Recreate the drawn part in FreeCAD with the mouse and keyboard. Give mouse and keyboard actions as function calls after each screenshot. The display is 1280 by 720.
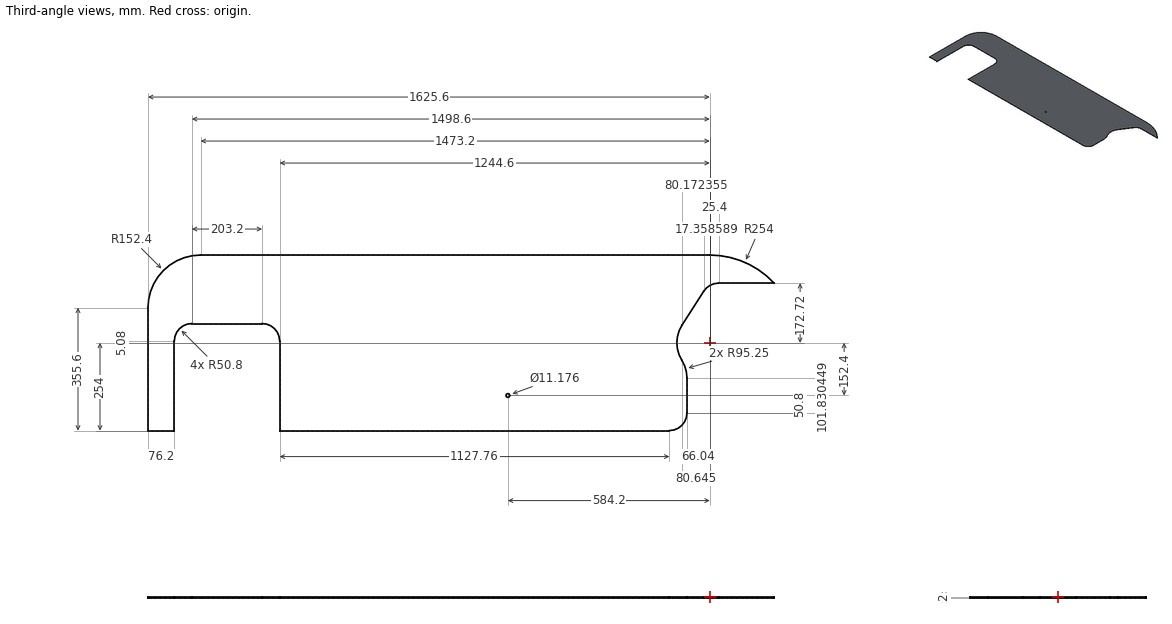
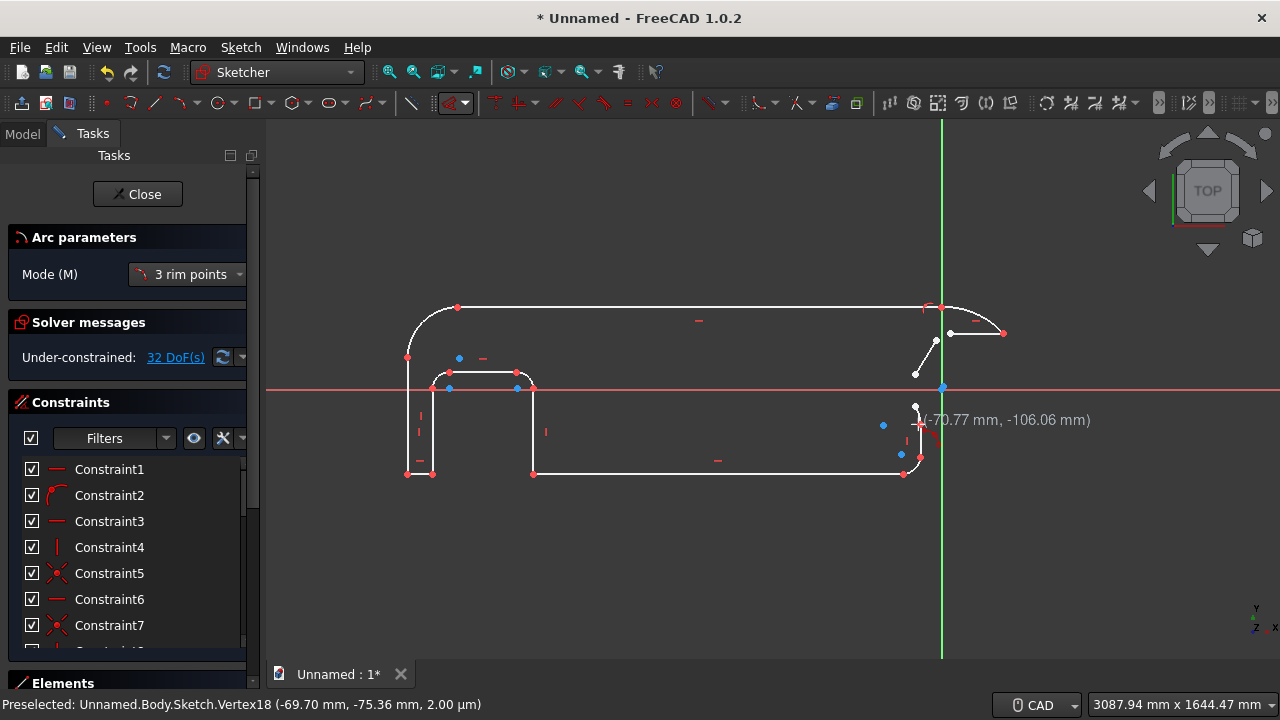
click(915, 407)
click(916, 374)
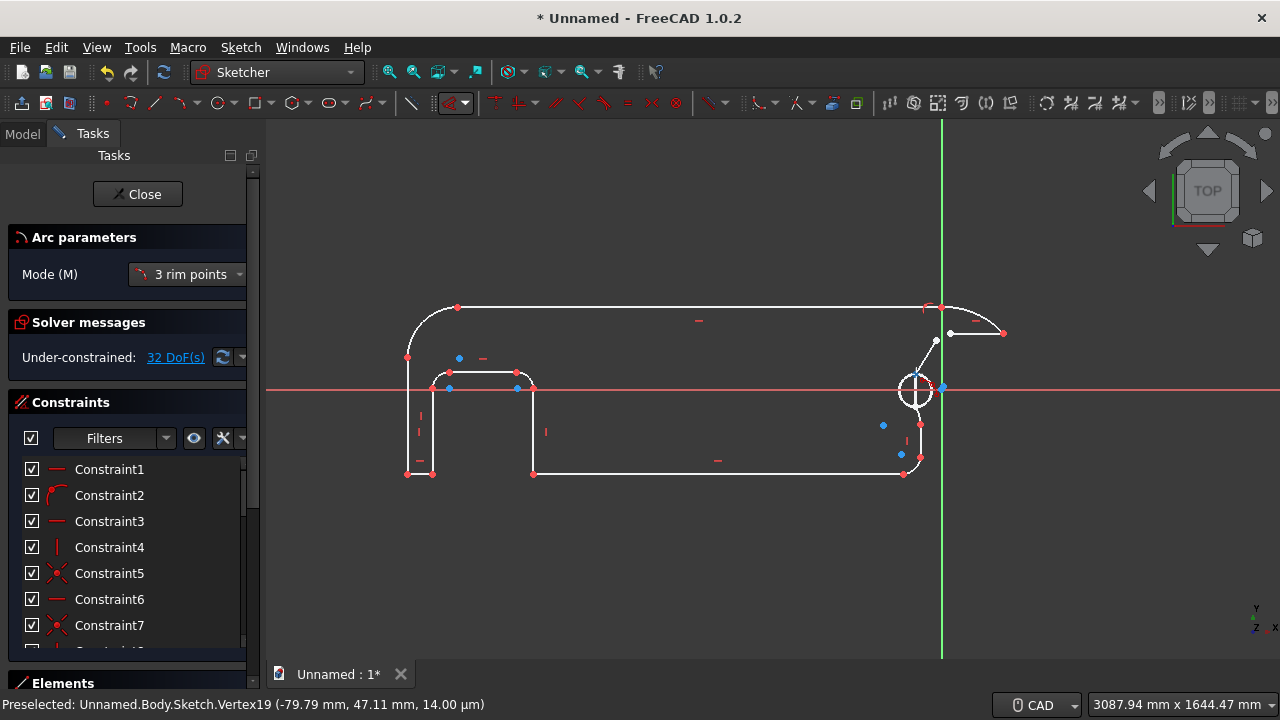
scroll(911, 397, up, 7)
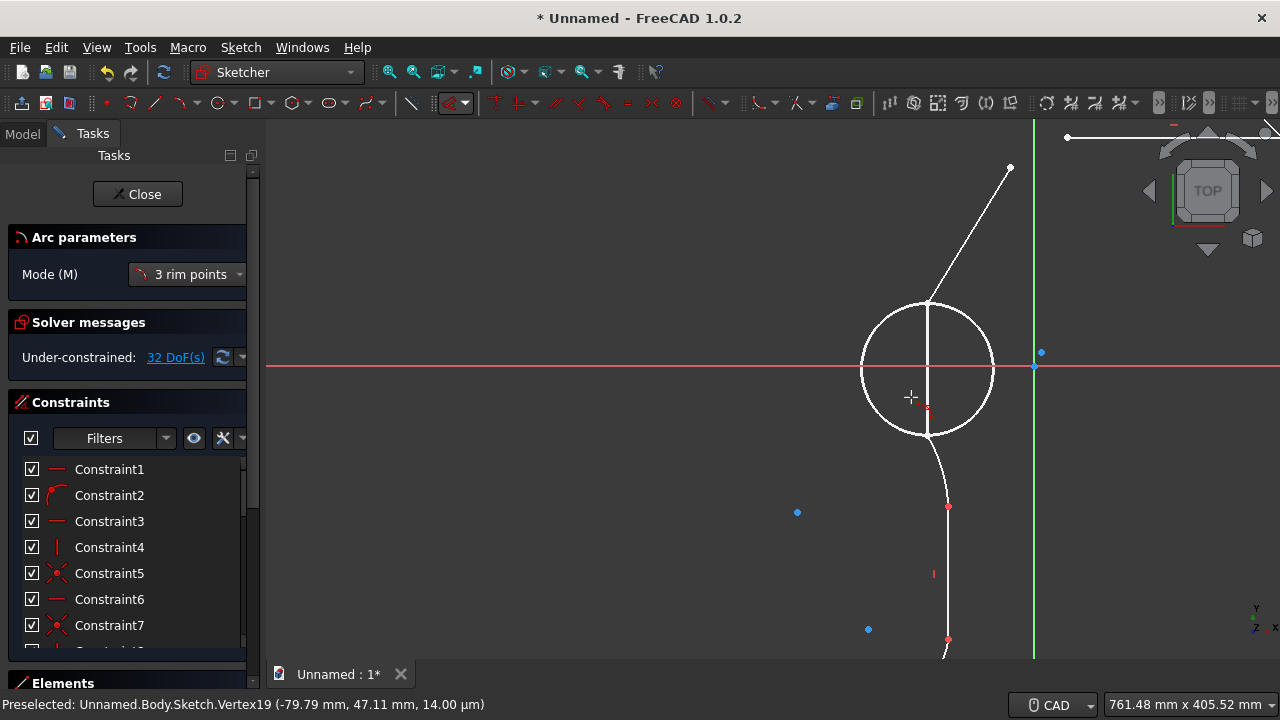
click(910, 394)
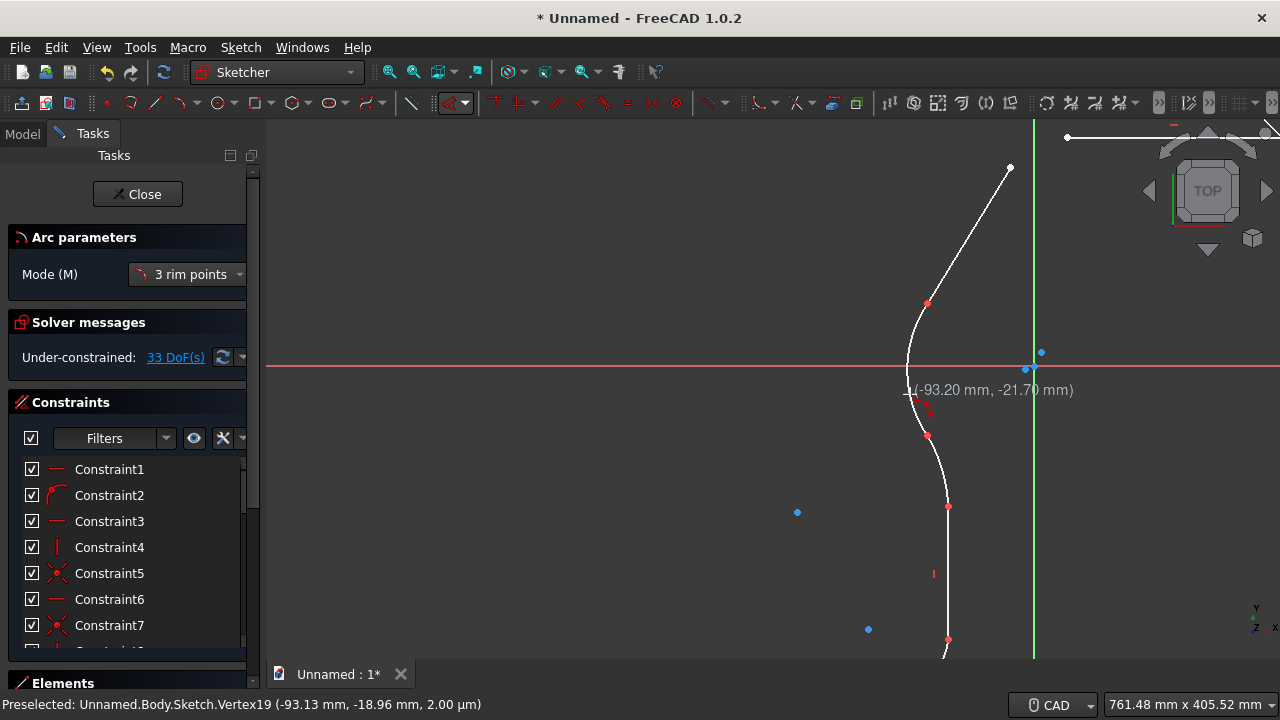
click(1011, 168)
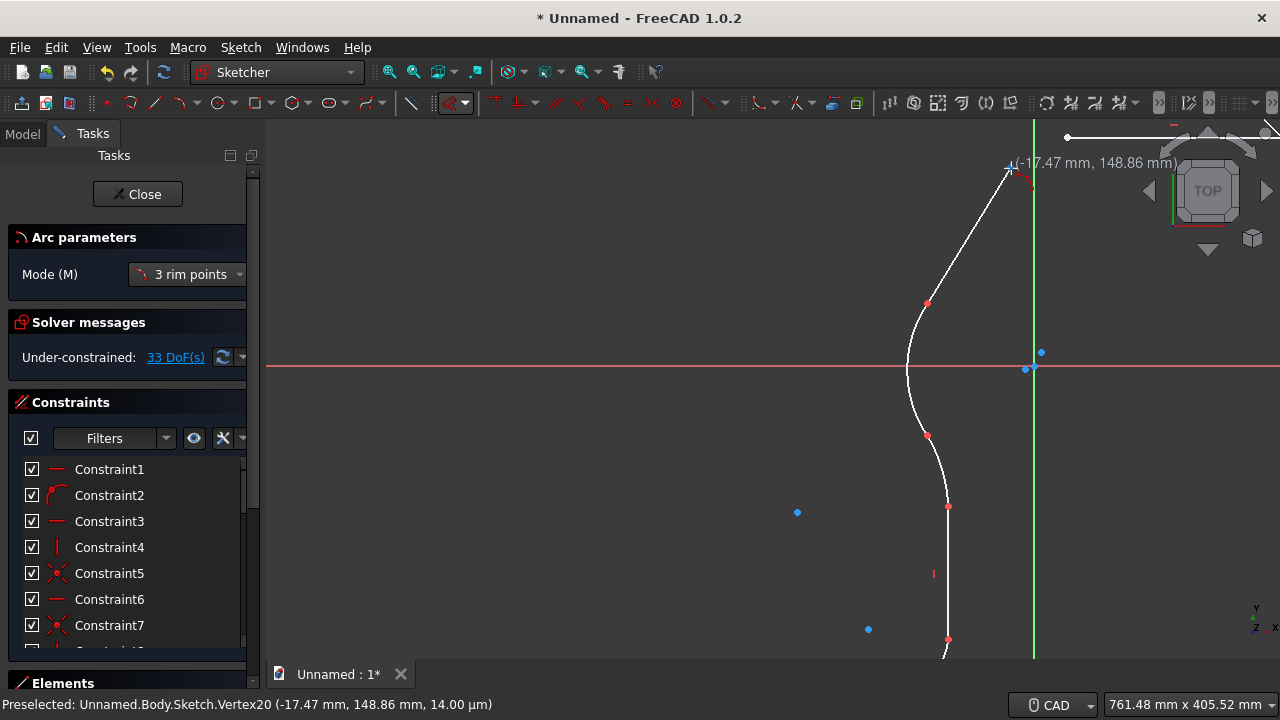
scroll(910, 396, down, 7)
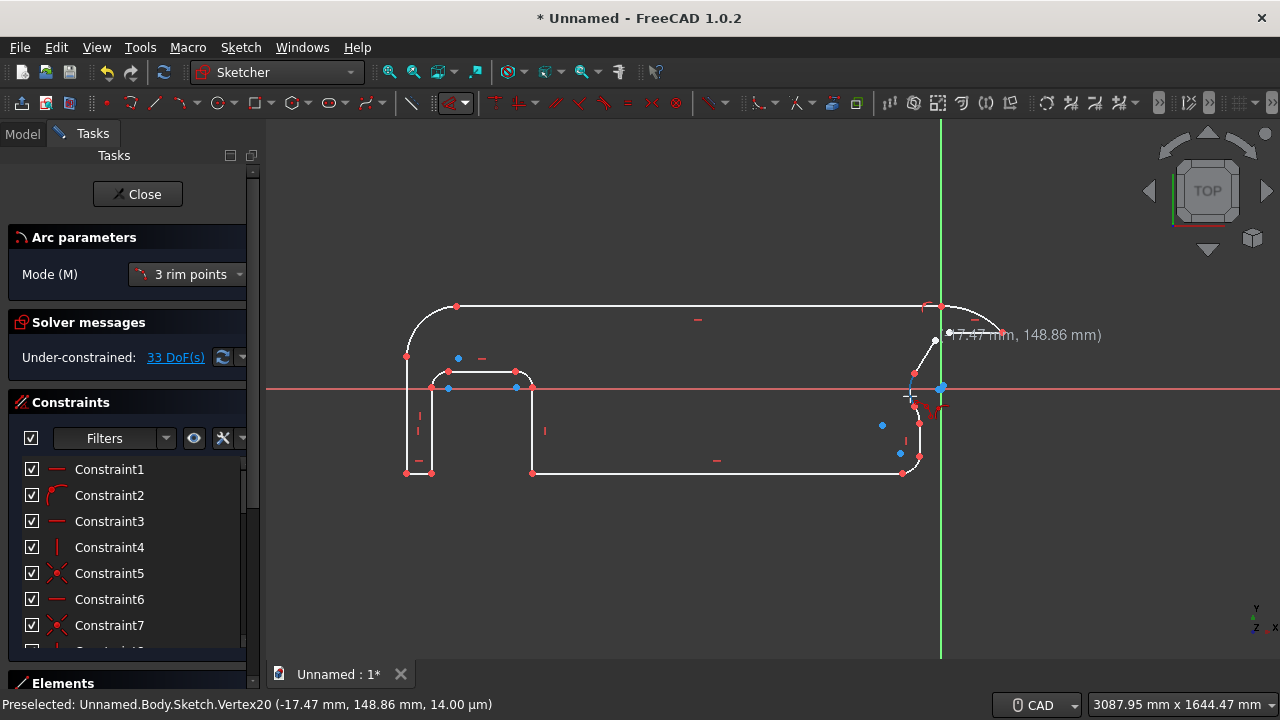
scroll(949, 332, up, 4)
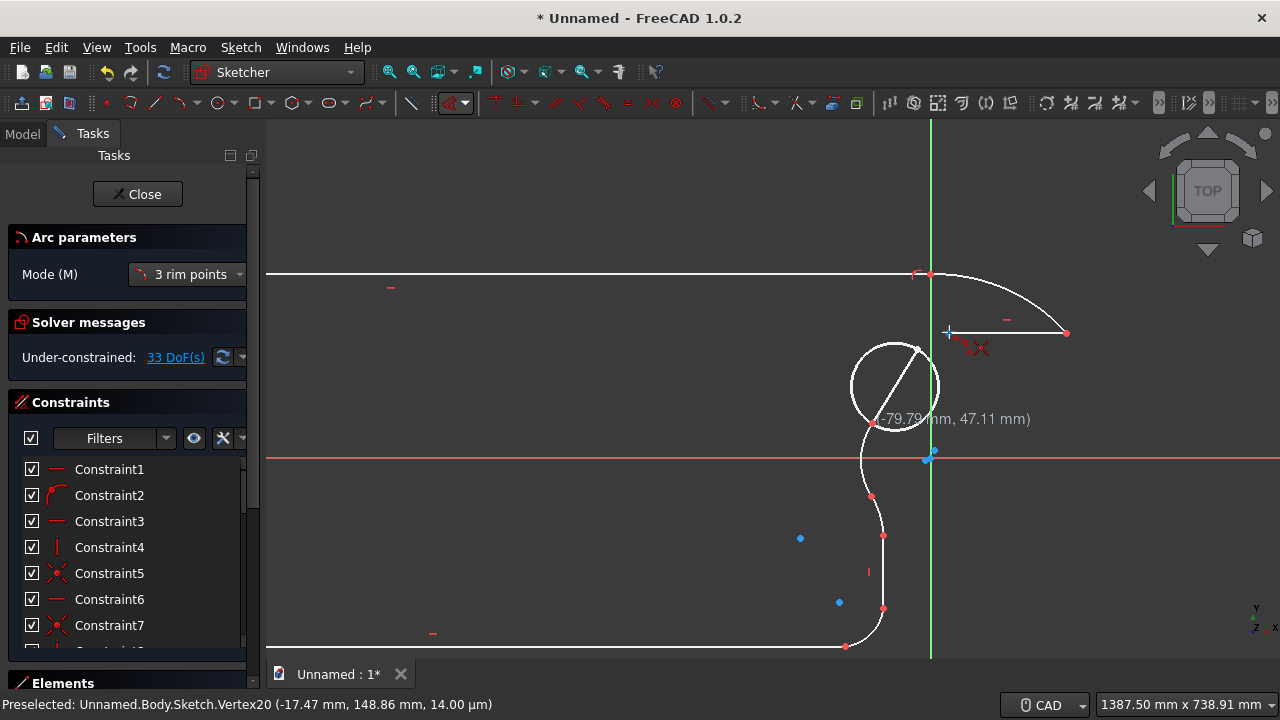
click(949, 333)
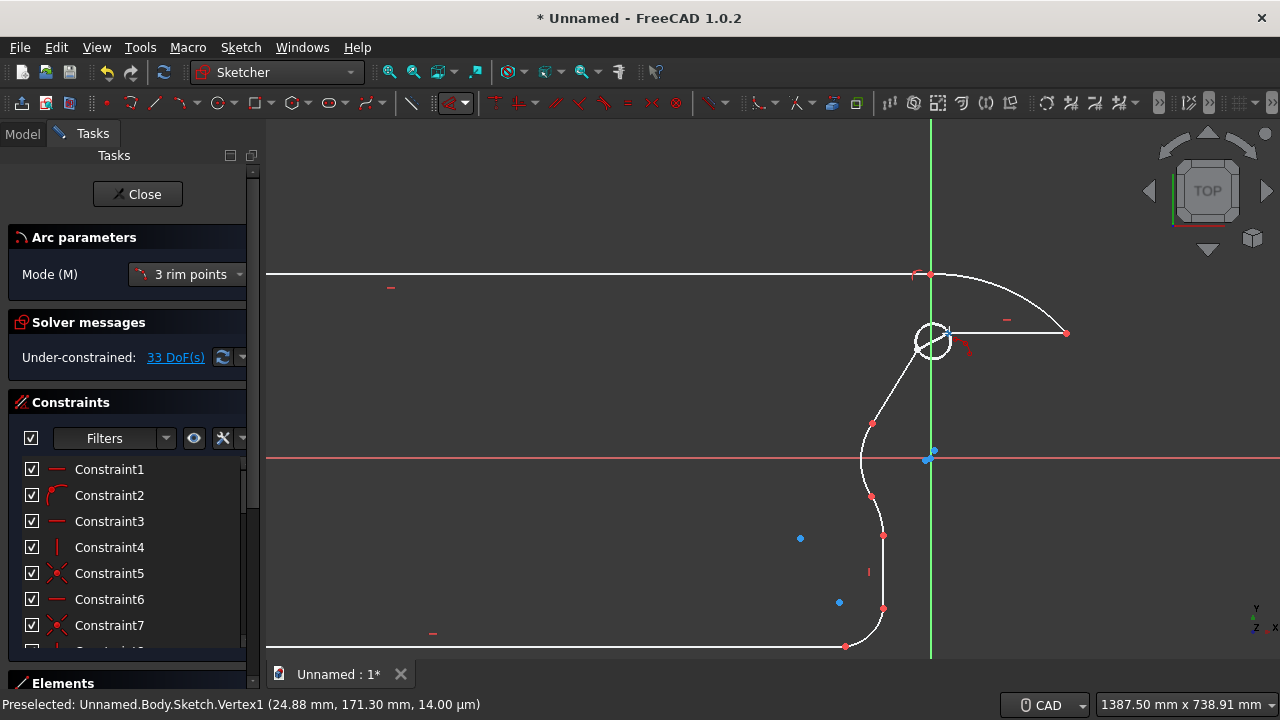
scroll(935, 335, up, 7)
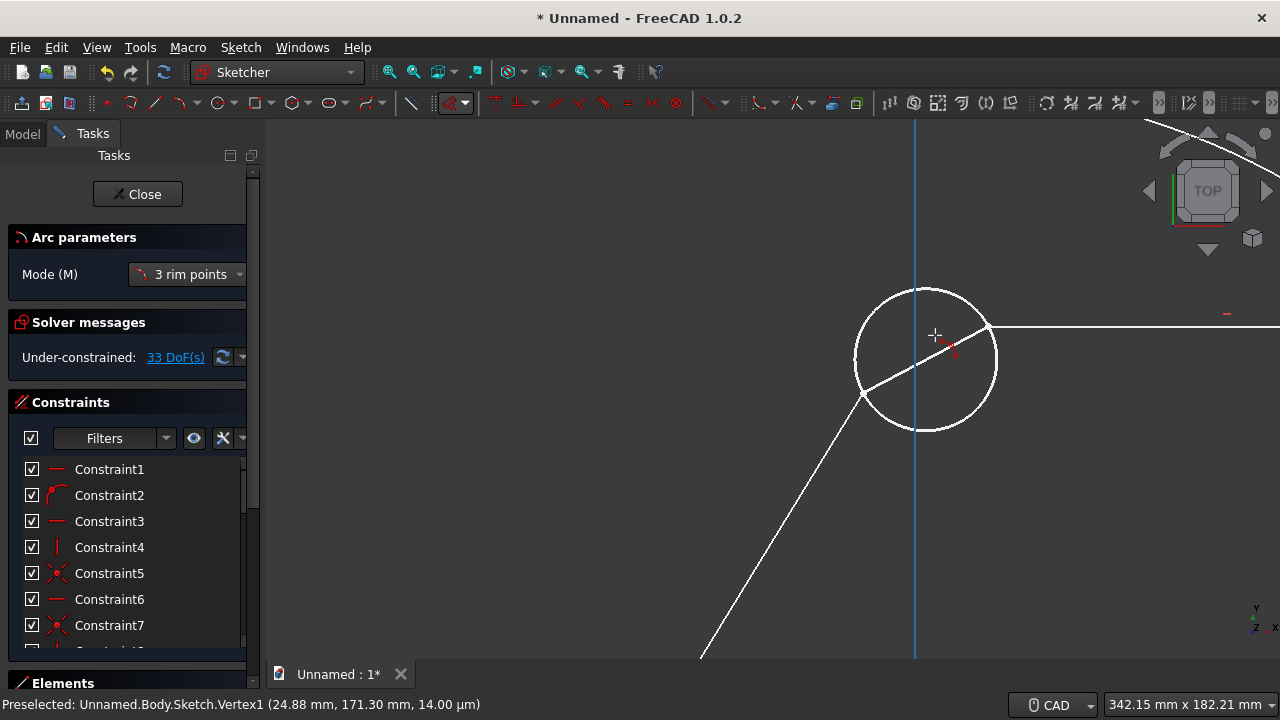
click(932, 334)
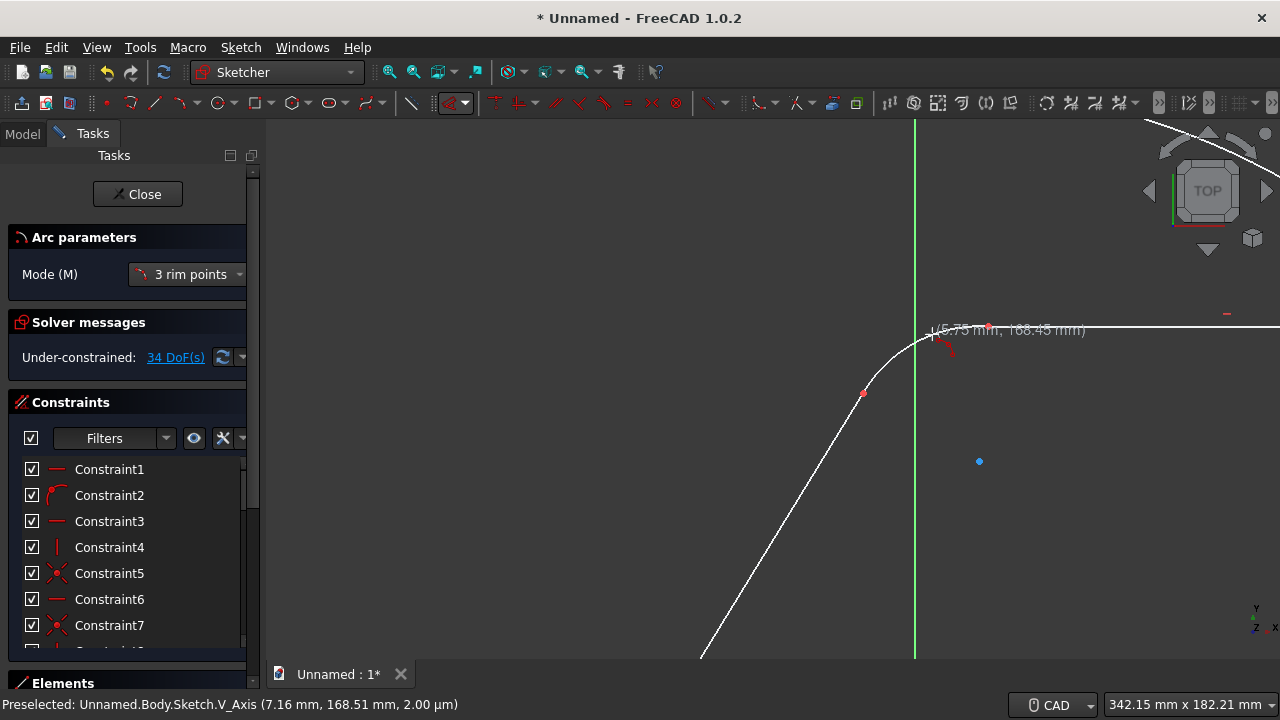
click(218, 104)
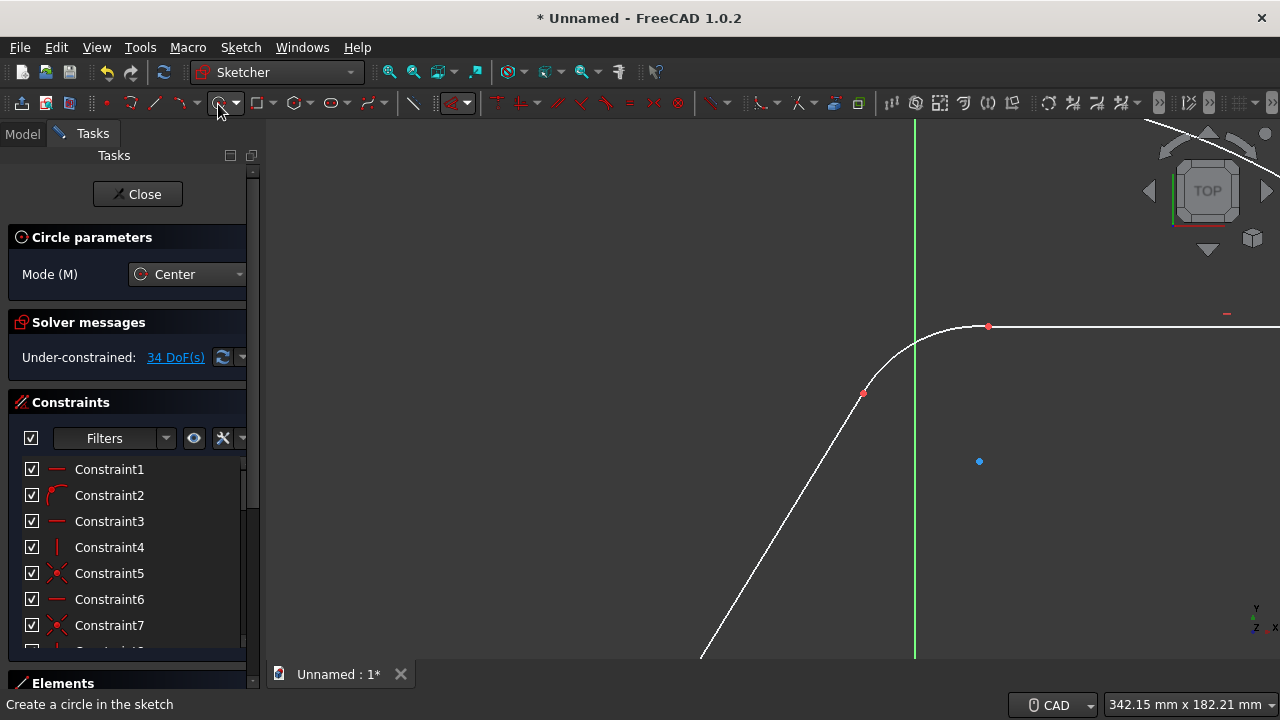
scroll(944, 334, down, 11)